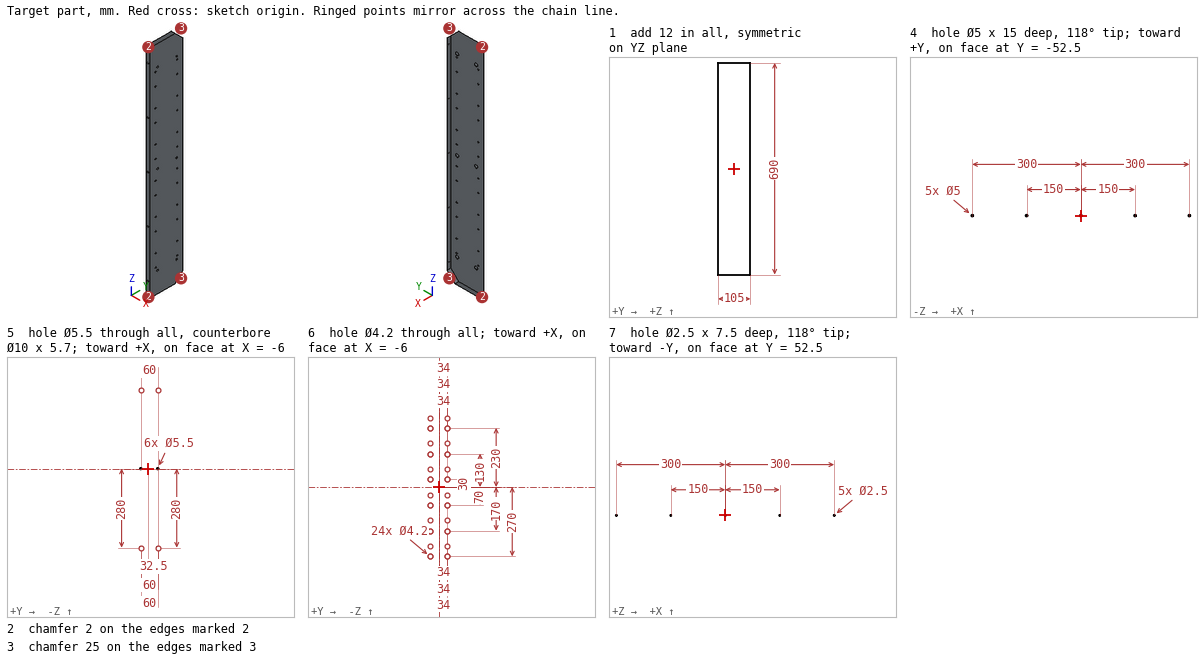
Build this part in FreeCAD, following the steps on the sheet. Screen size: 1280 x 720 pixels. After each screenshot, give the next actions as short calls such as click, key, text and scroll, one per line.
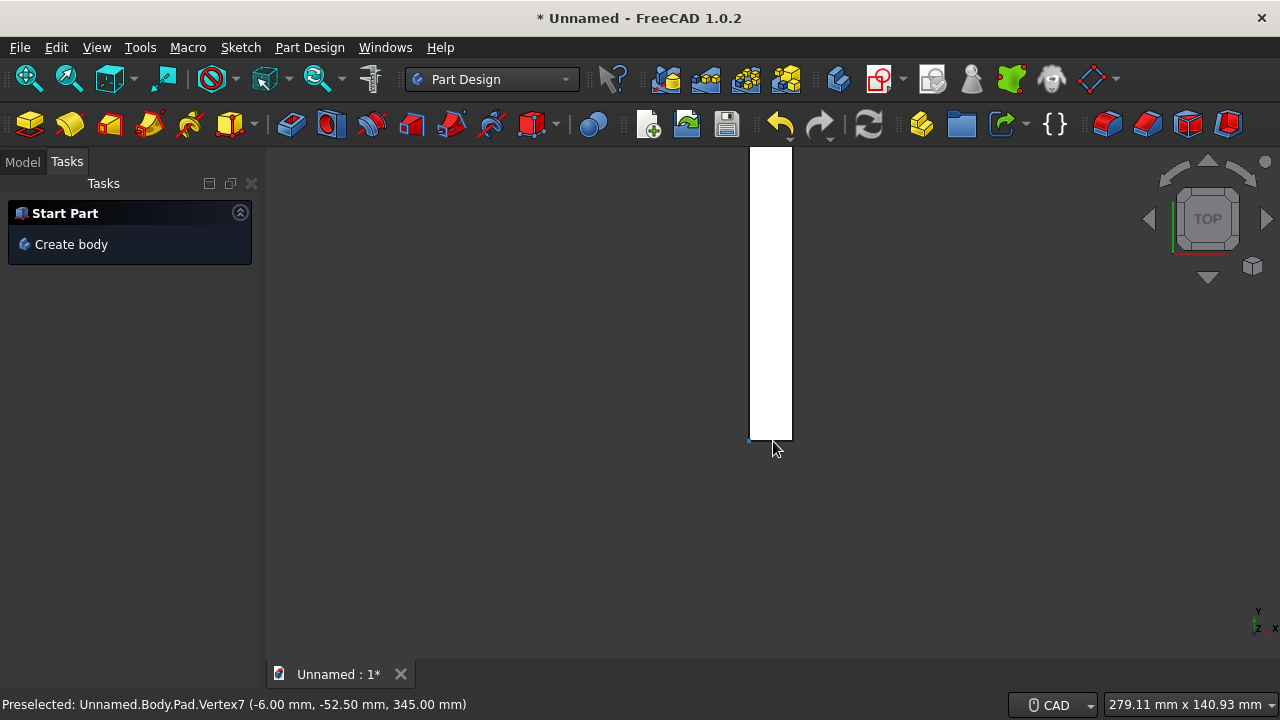
click(771, 440)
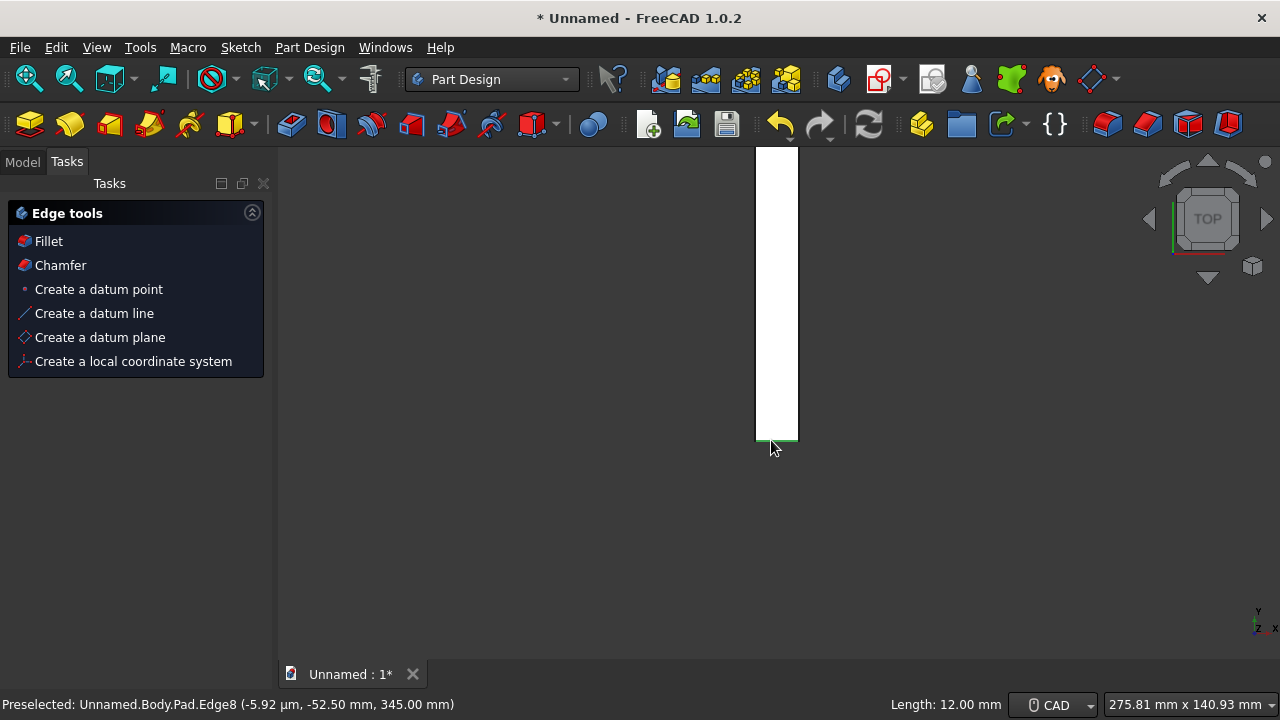
click(30, 80)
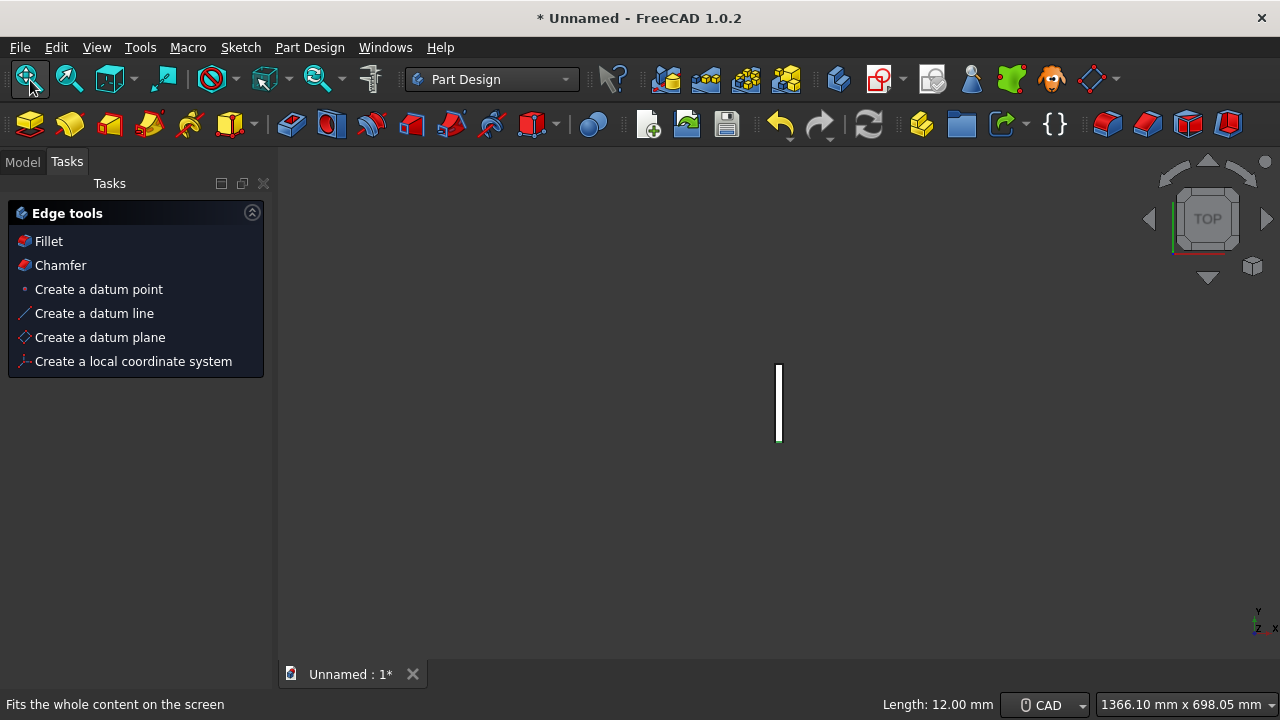
key(1)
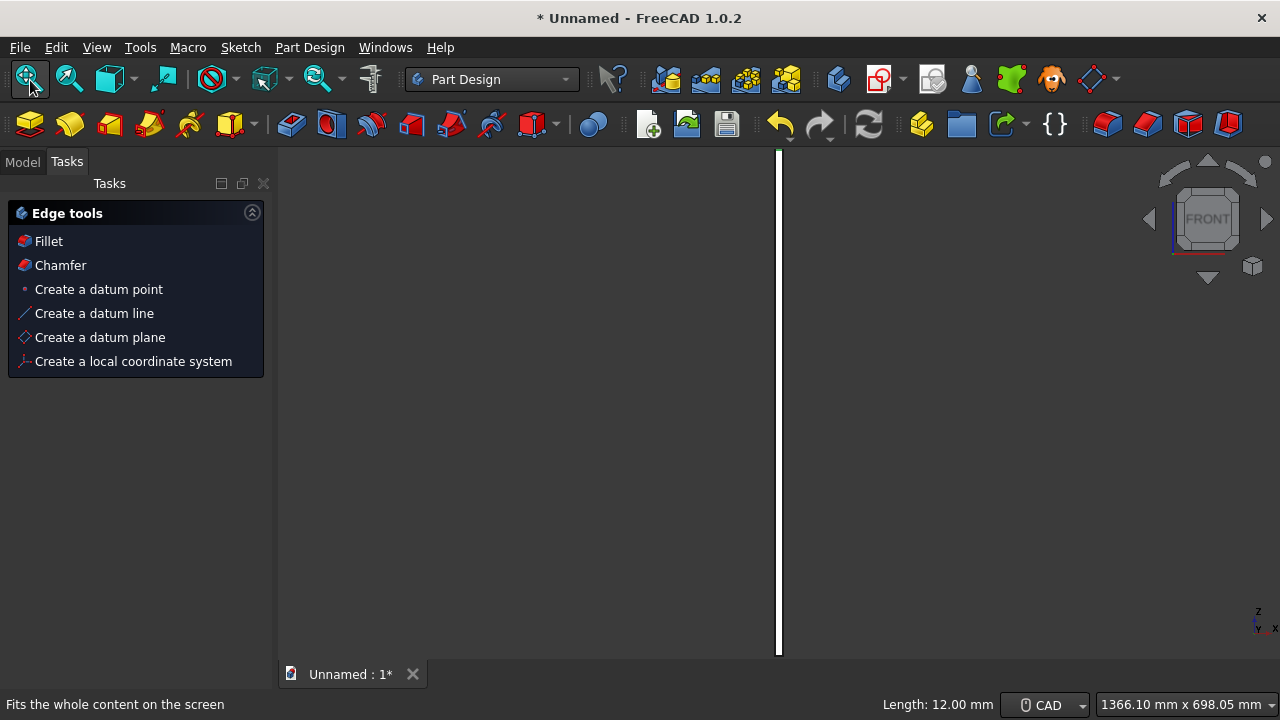
key(3)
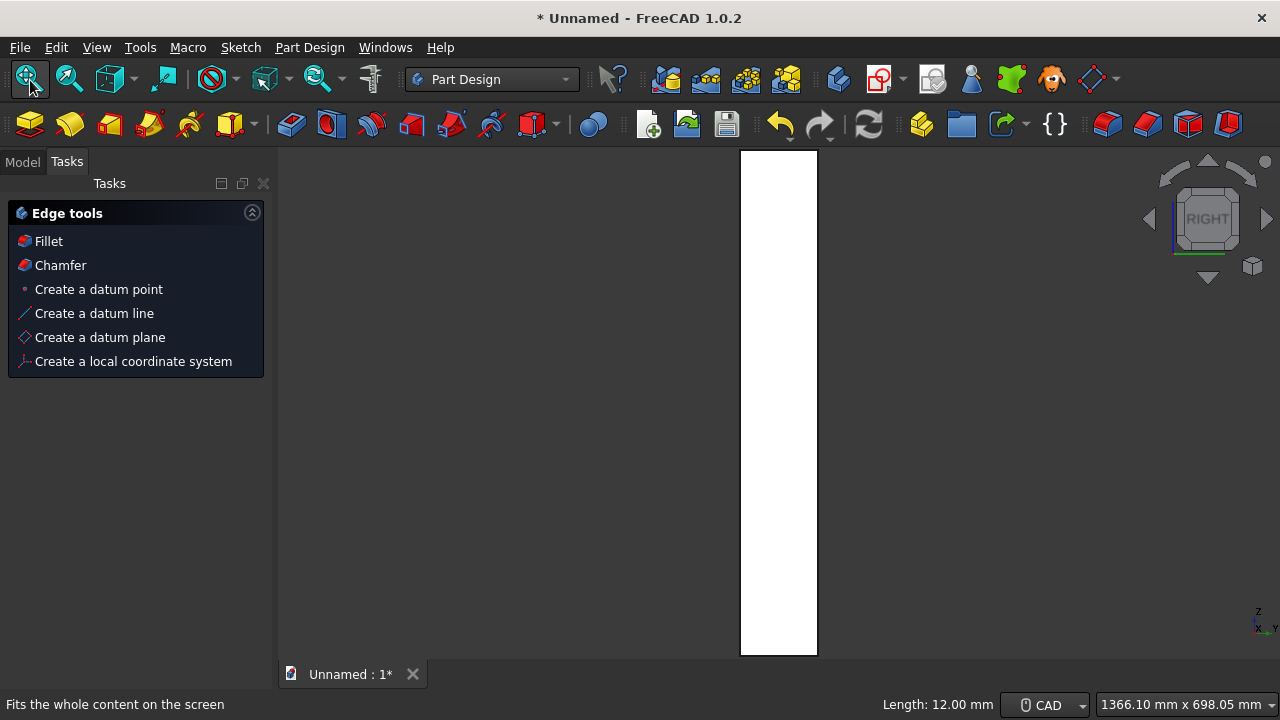
key(5)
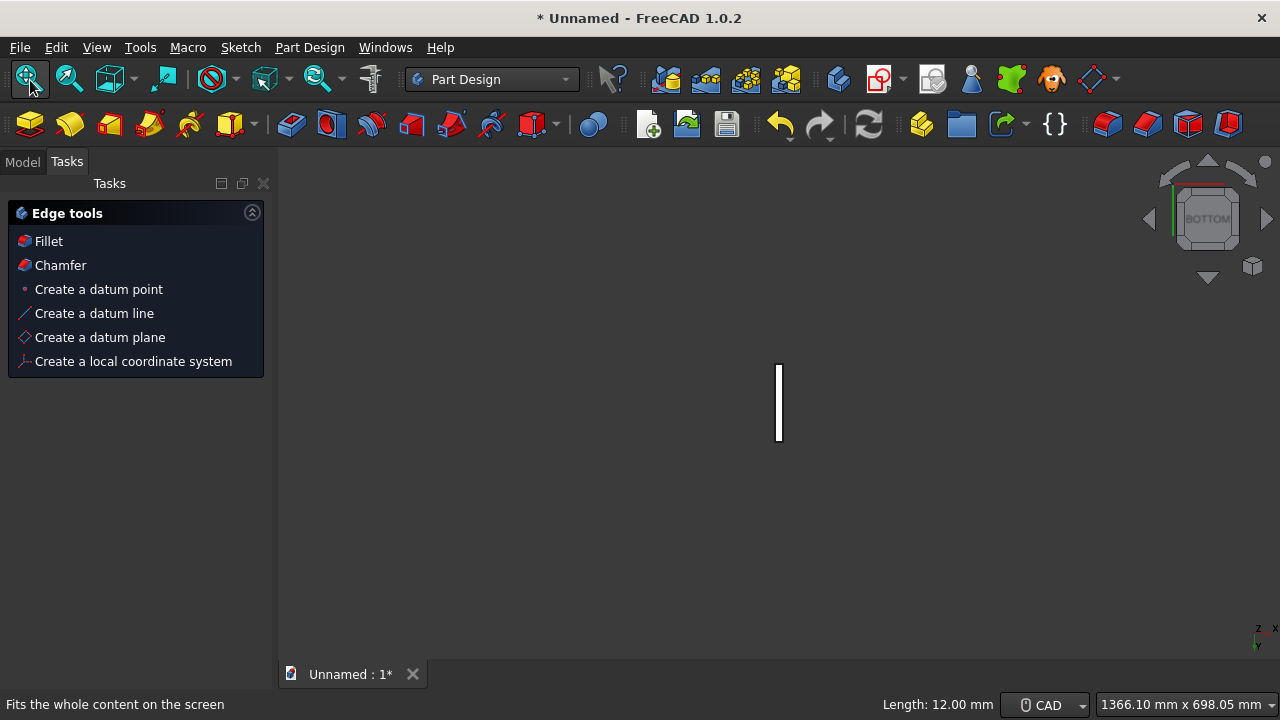
click(30, 80)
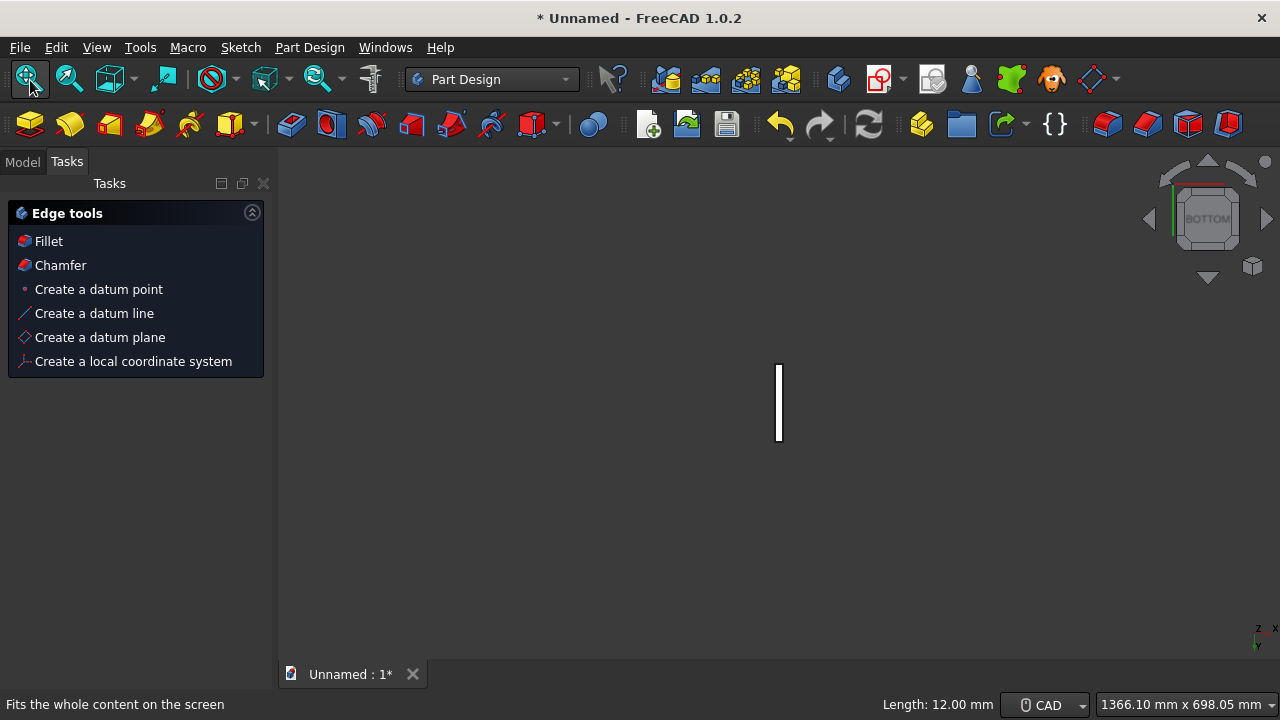
scroll(779, 363, up, 8)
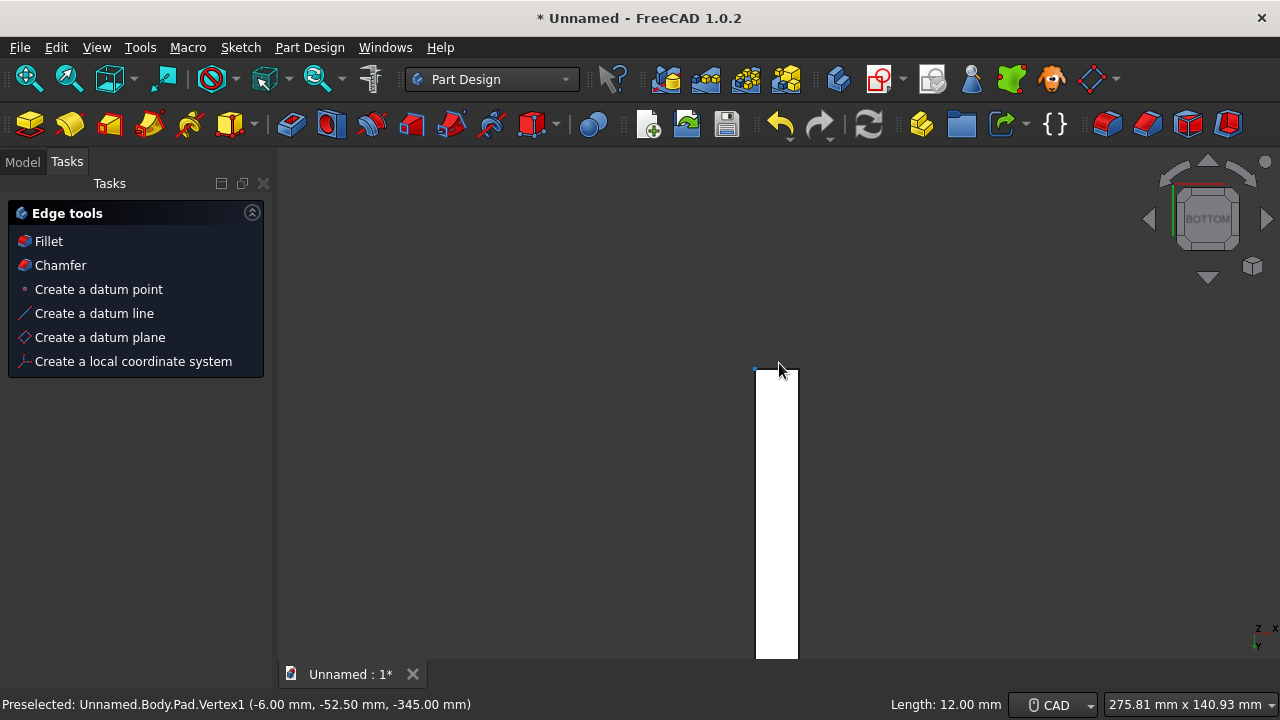
click(777, 368, ctrl)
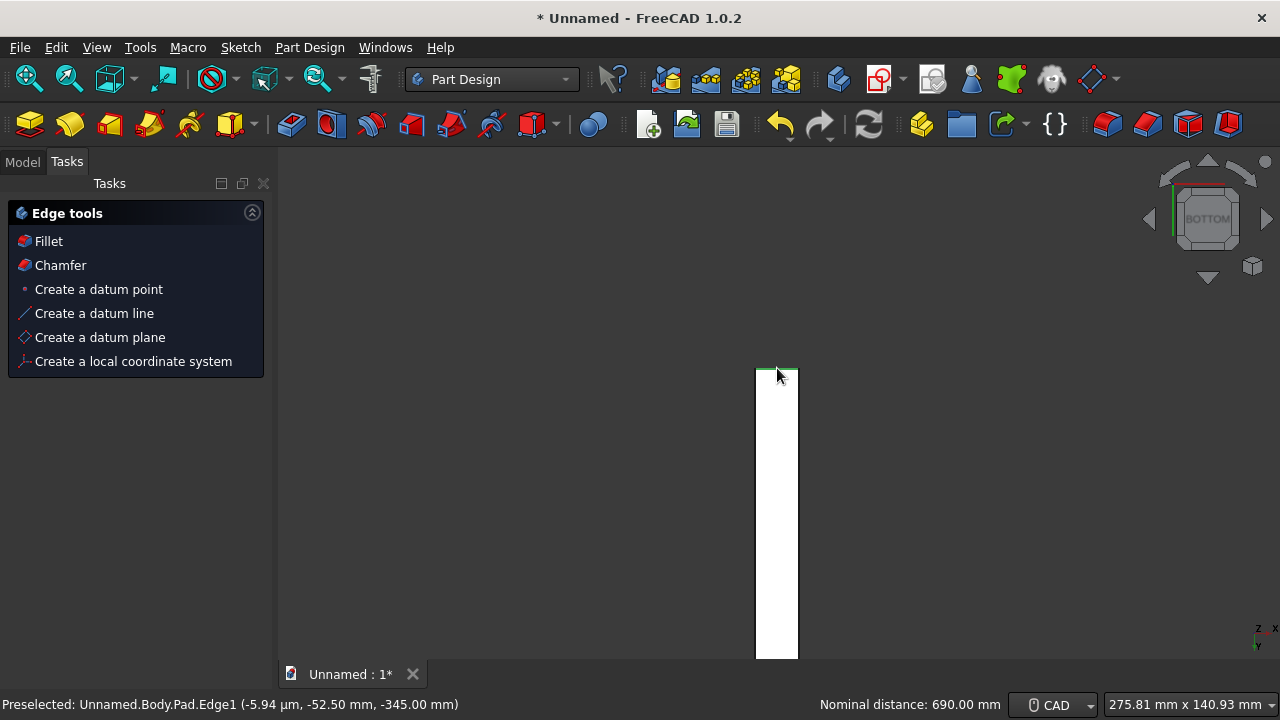
click(1148, 124)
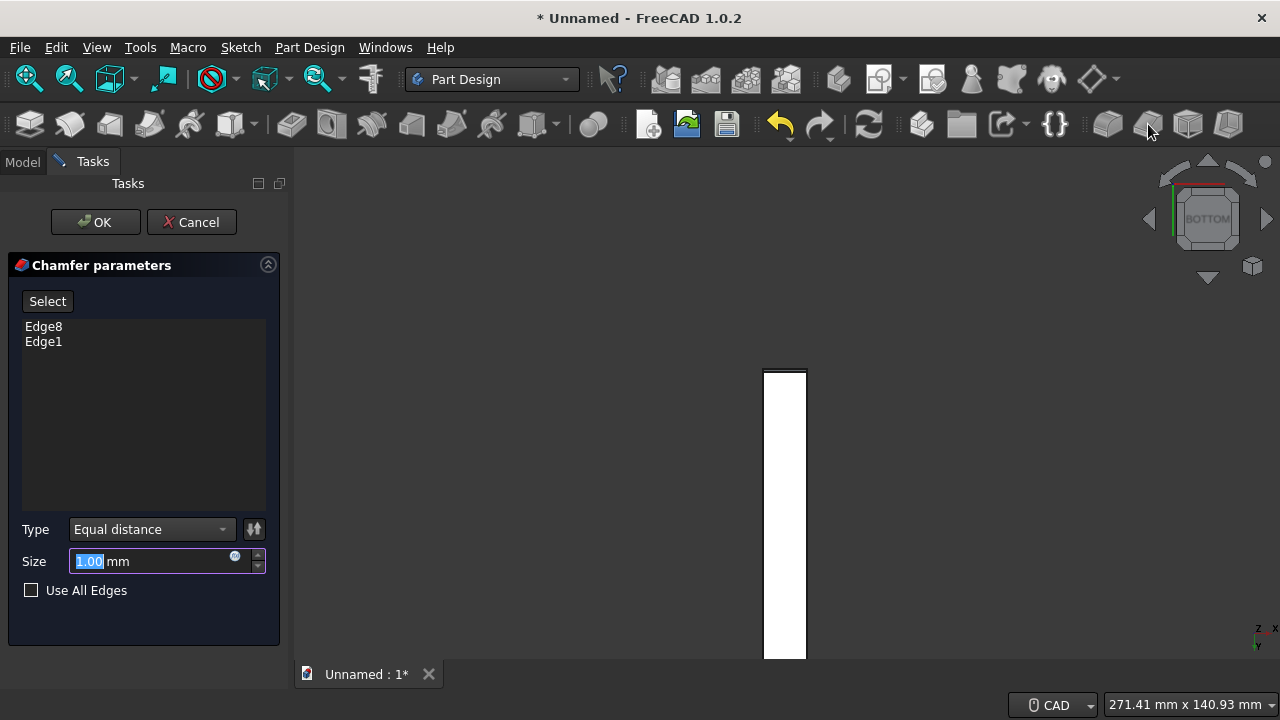
text(2)
key(Tab)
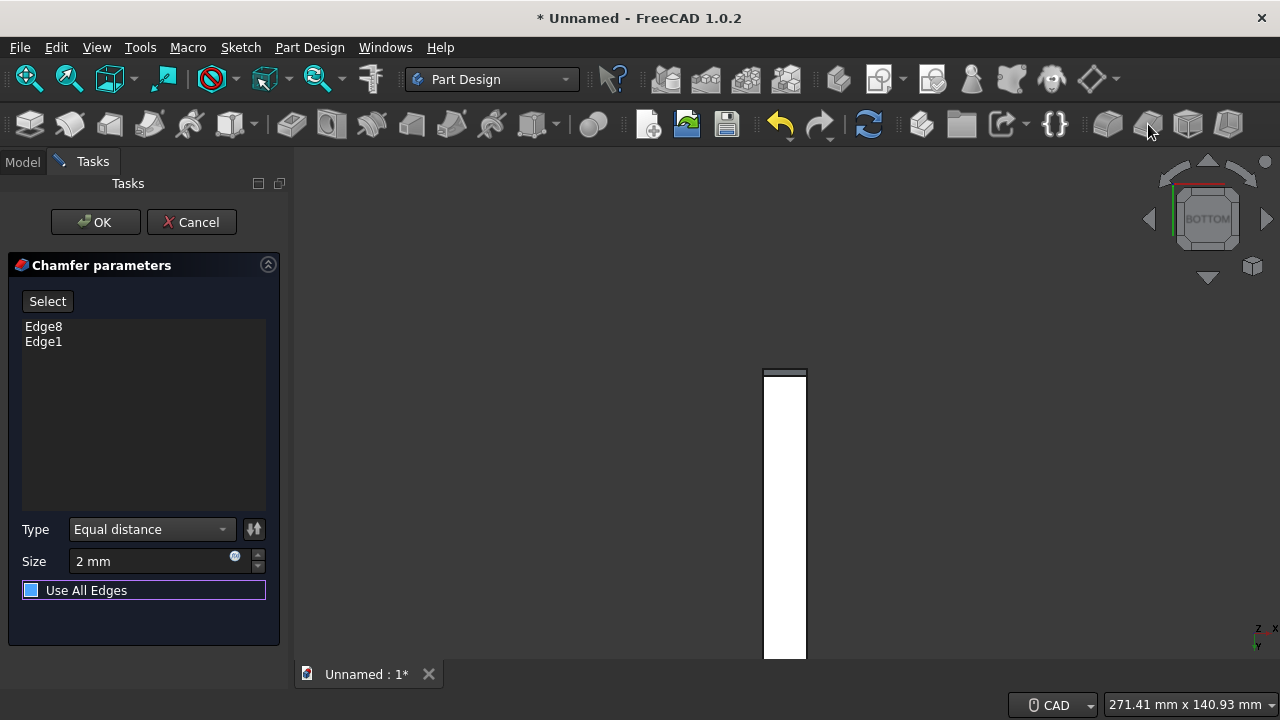
click(96, 222)